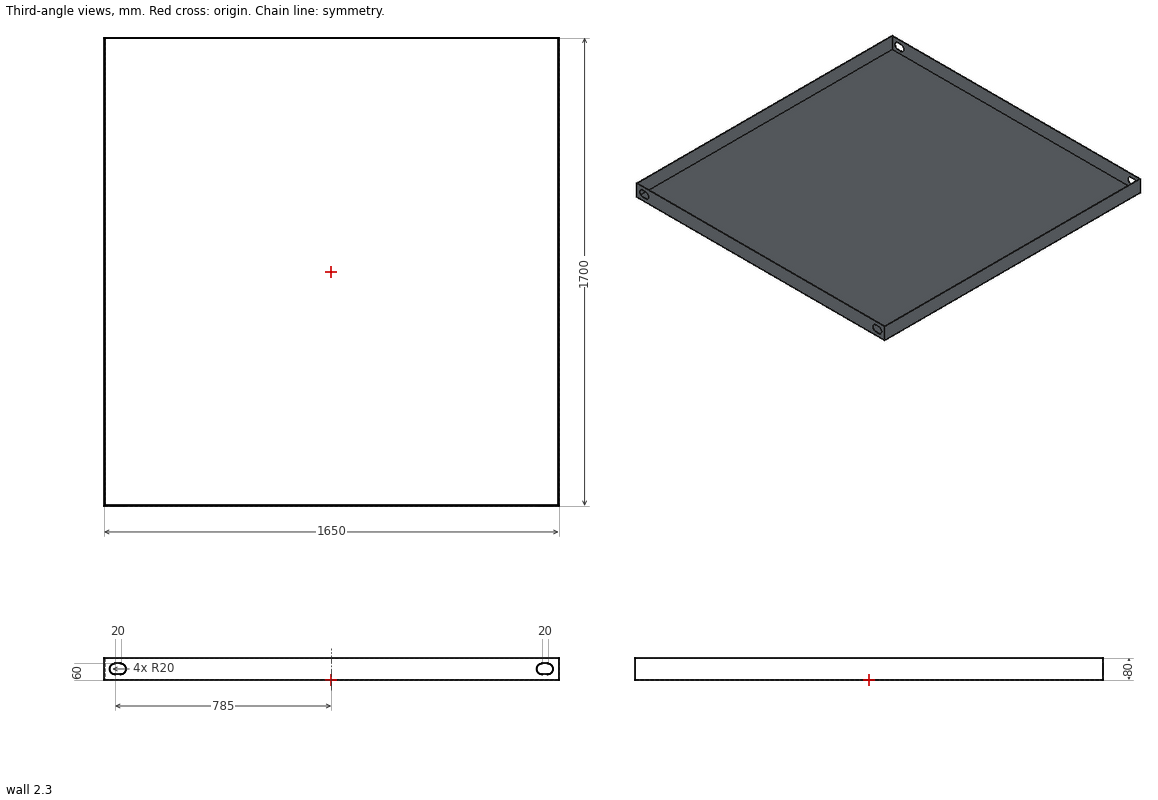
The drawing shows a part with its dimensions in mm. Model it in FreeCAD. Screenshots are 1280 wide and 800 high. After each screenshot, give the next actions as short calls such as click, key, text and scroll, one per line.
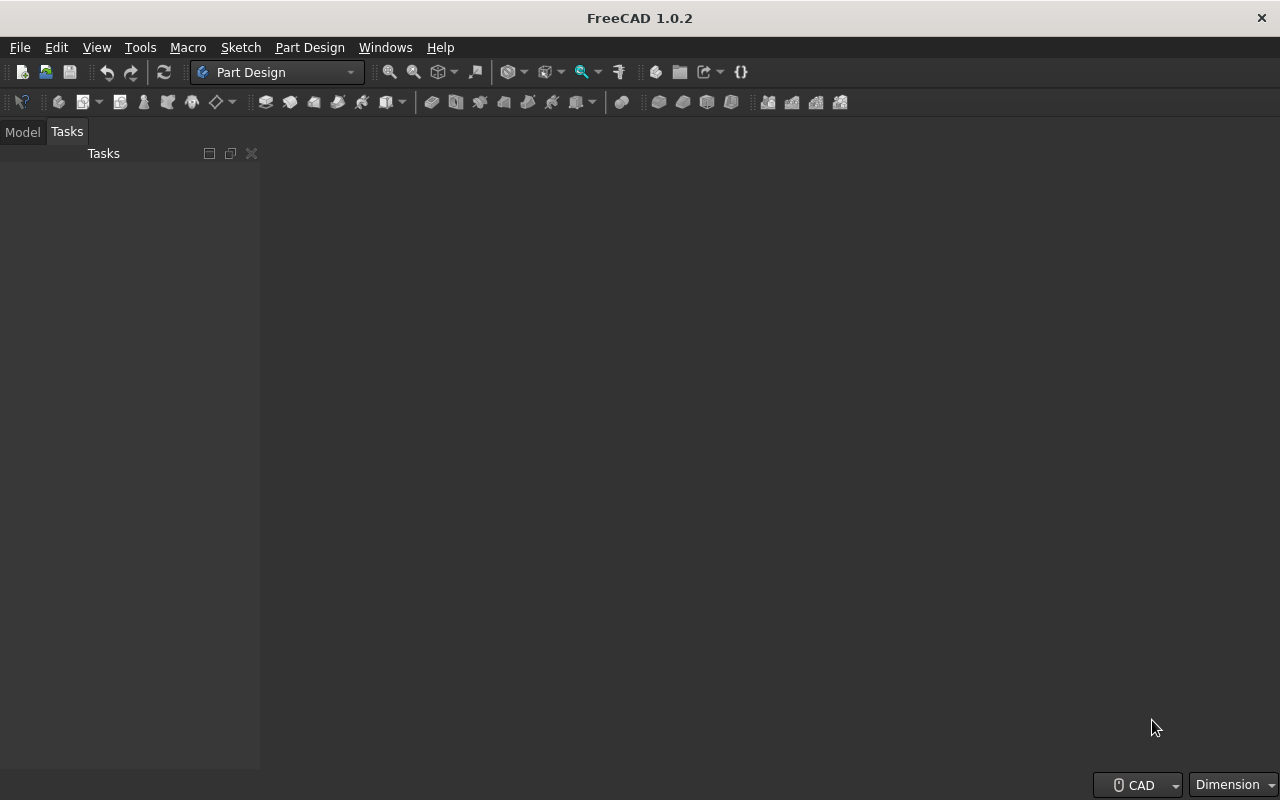
key(ctrl+n)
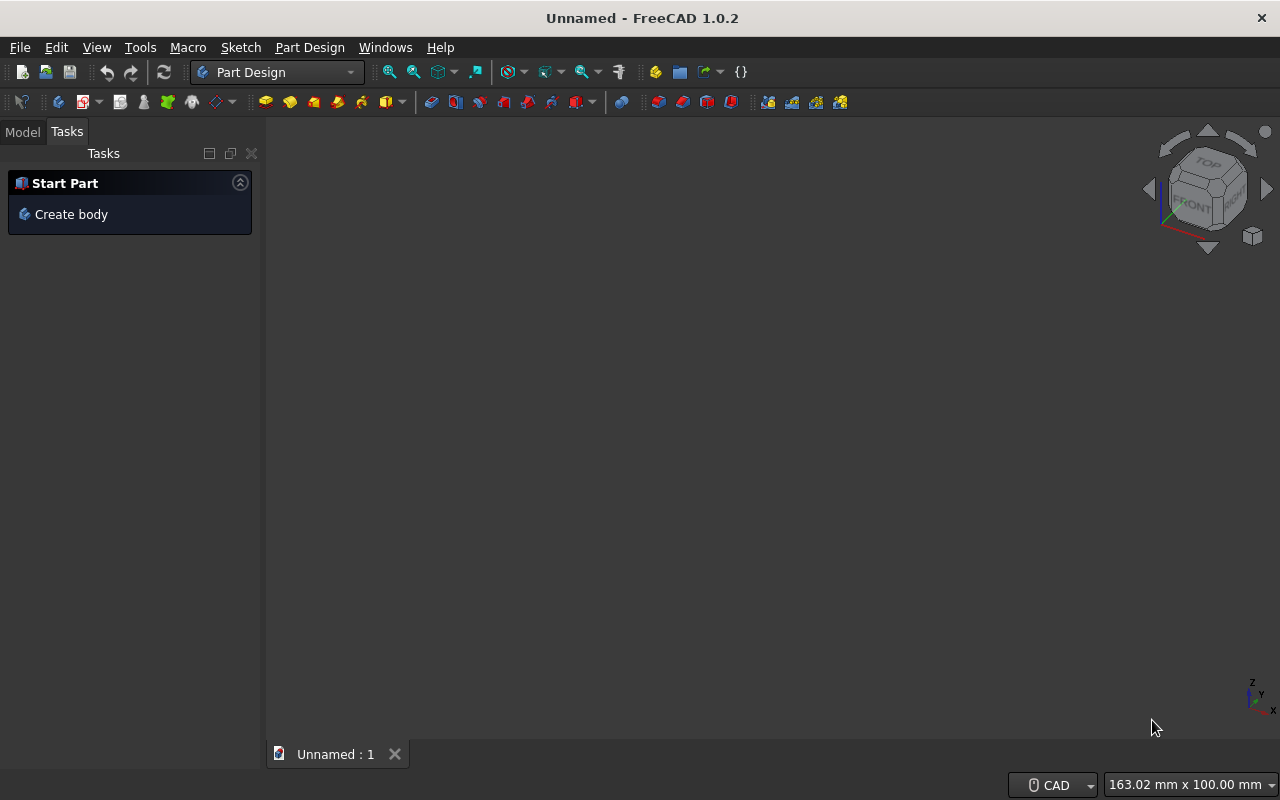
click(84, 102)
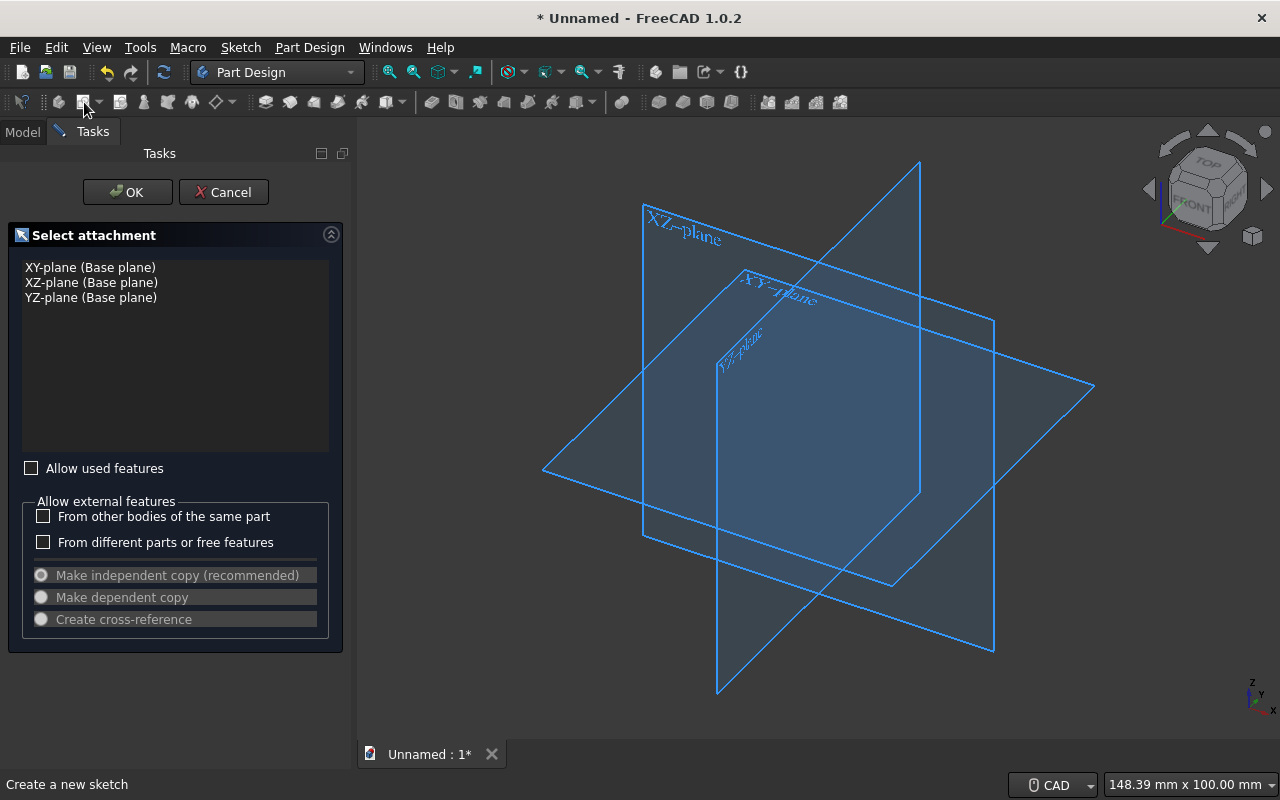
click(82, 268)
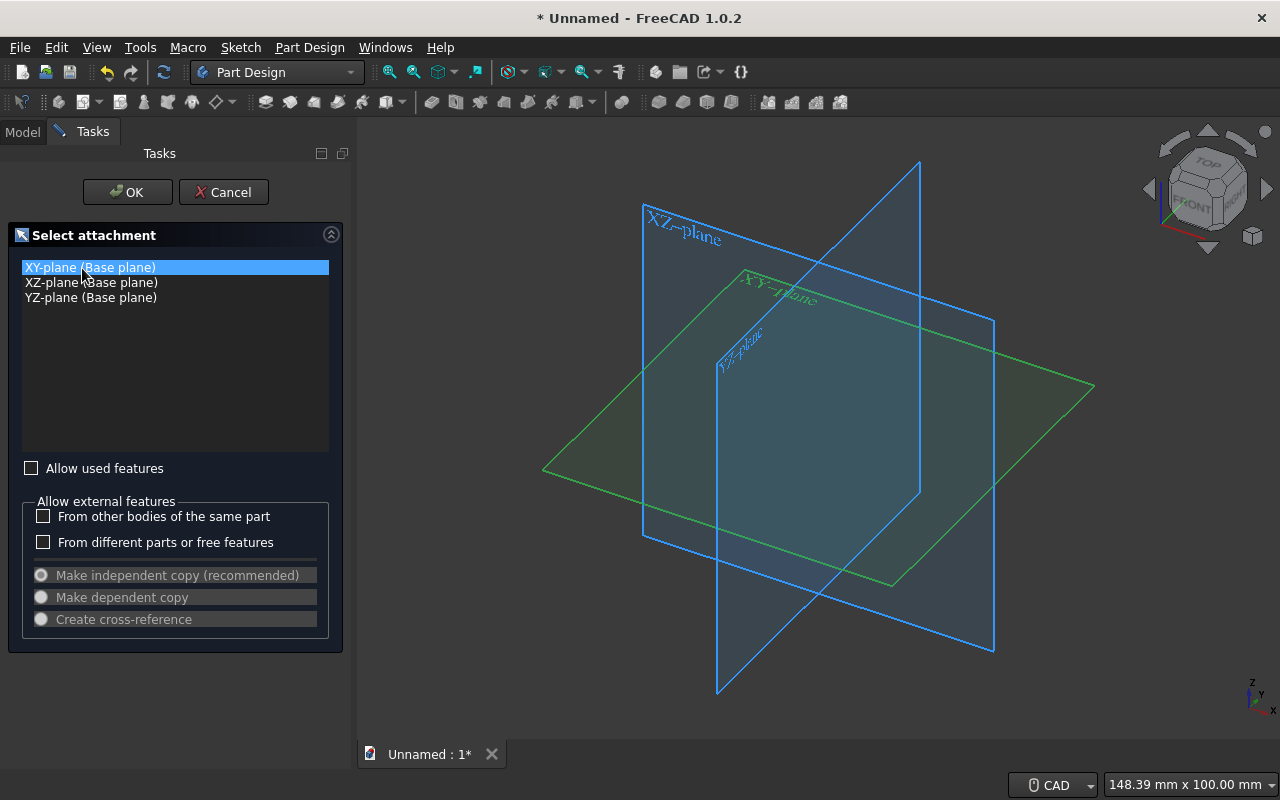
click(128, 192)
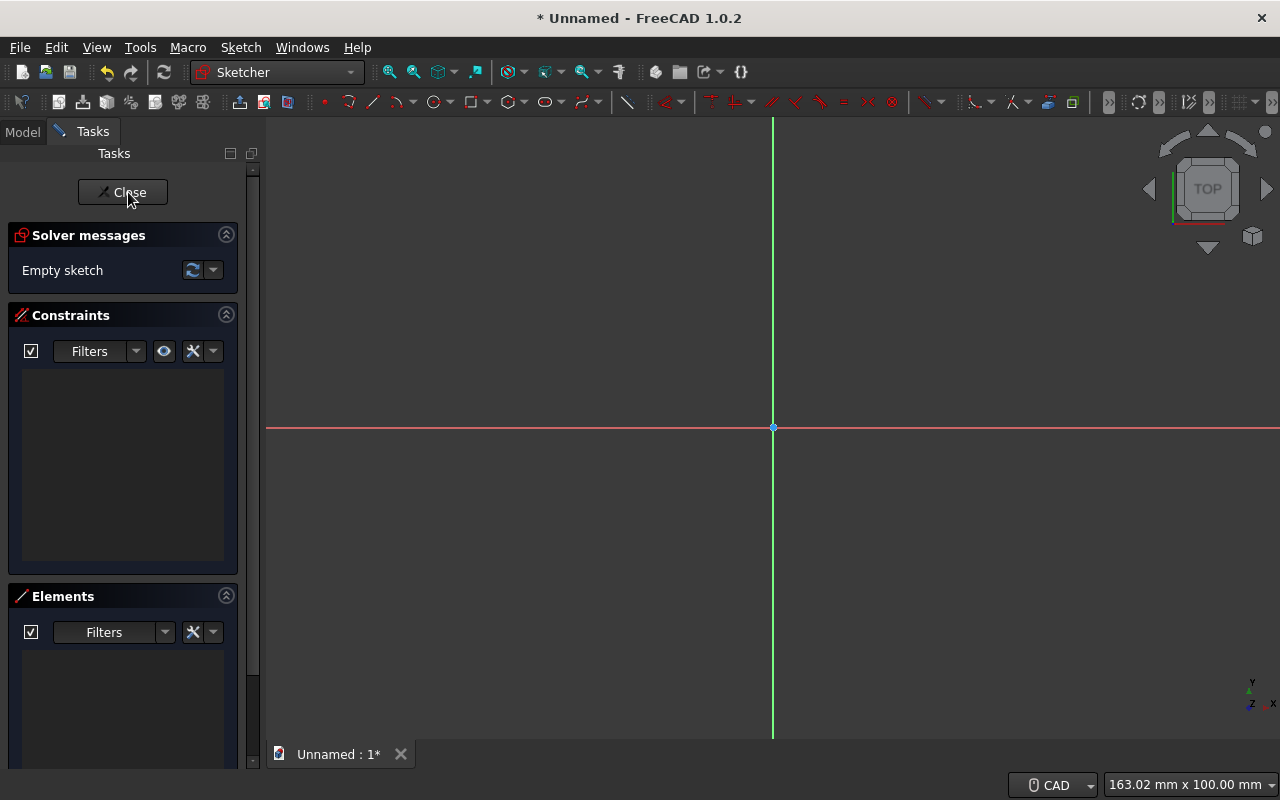
scroll(702, 428, down, 16)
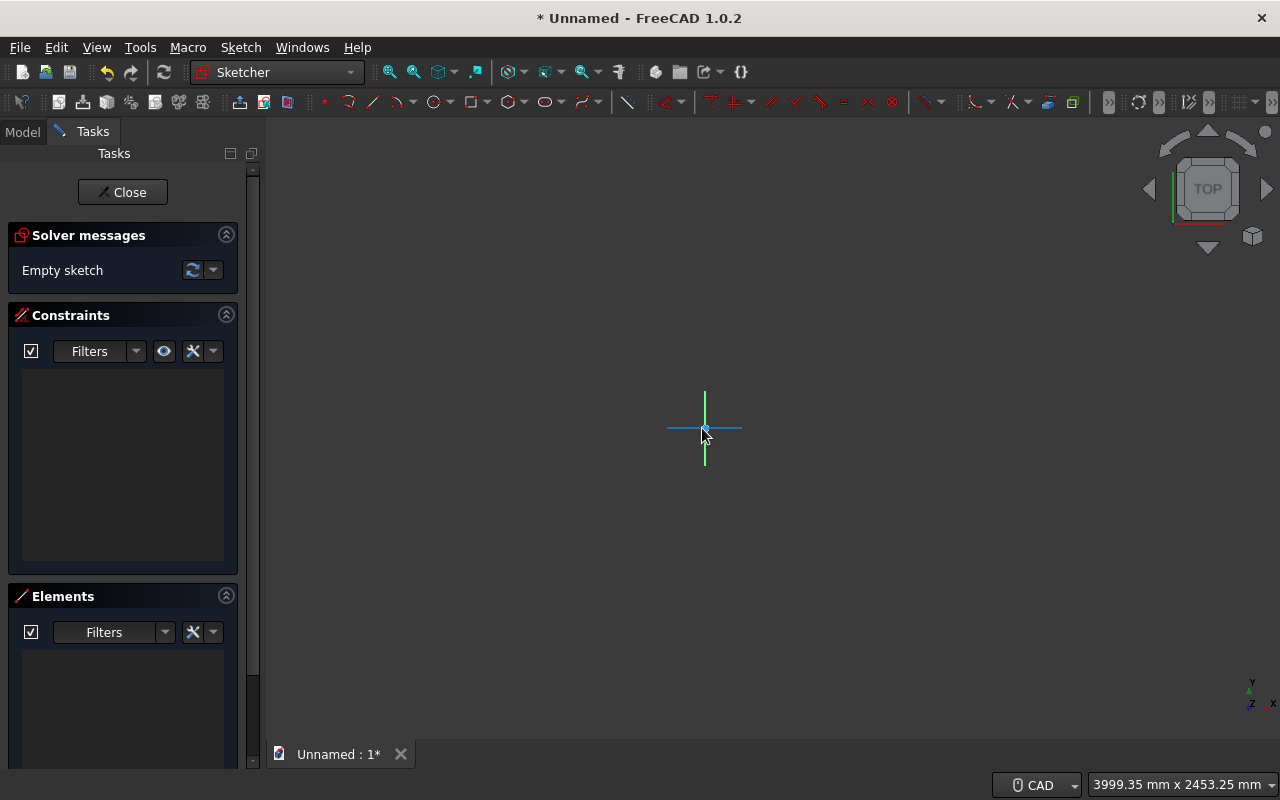
key(g)
key(v)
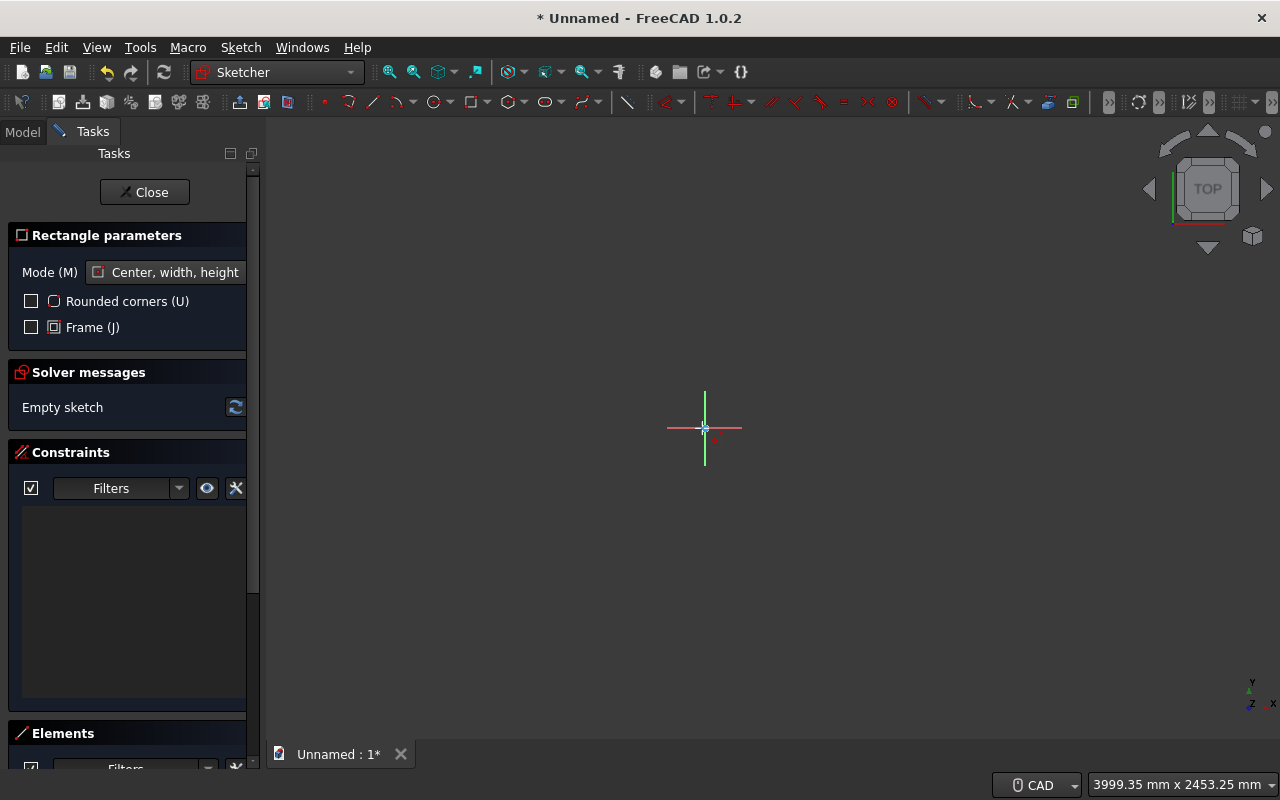
click(705, 428)
move(914, 213)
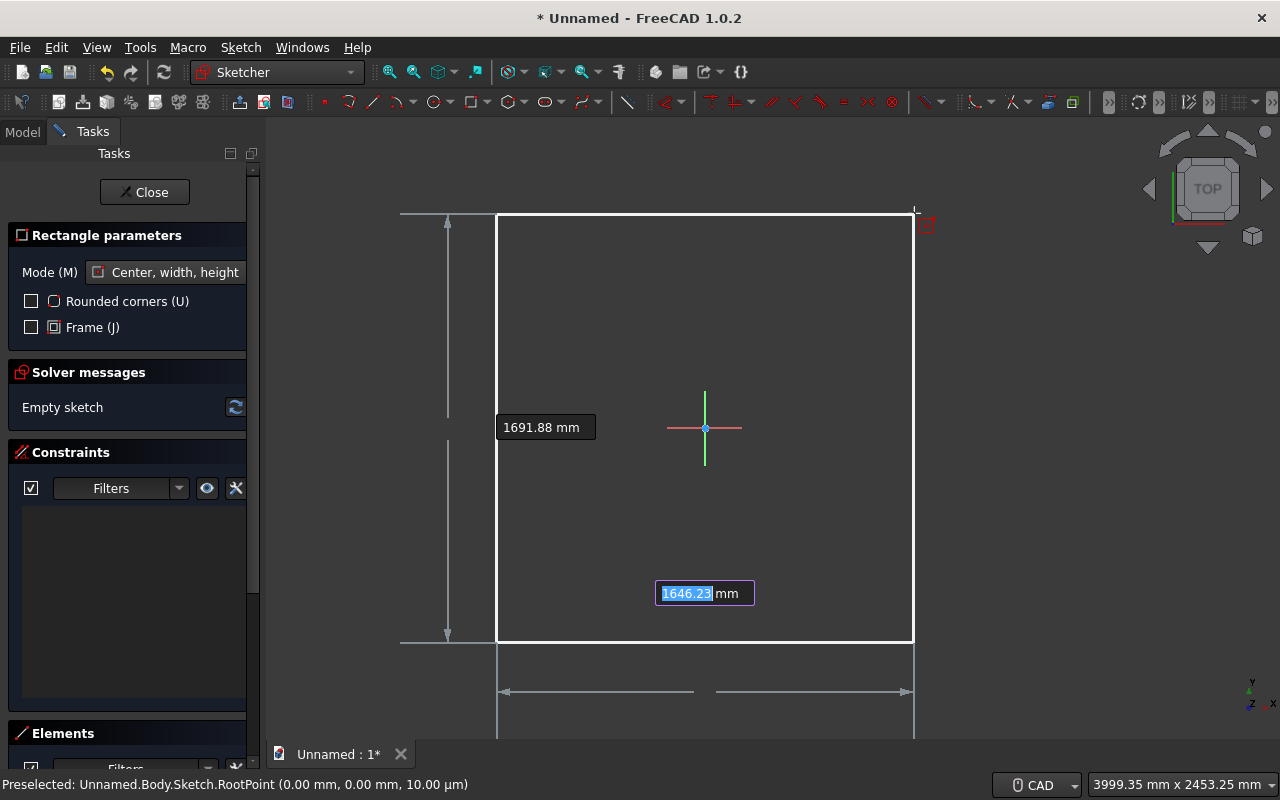
text(1650)
key(Tab)
text(1700)
key(Return)
key(Escape)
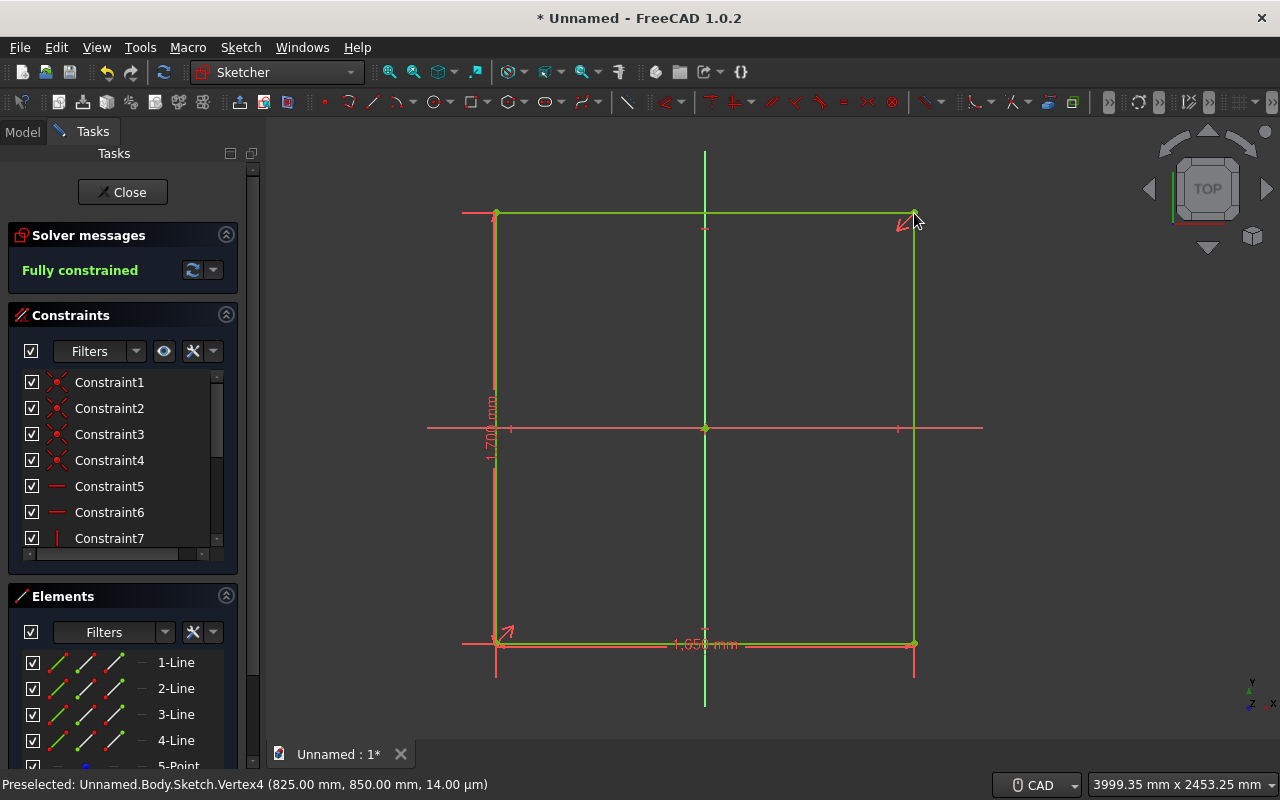
click(123, 192)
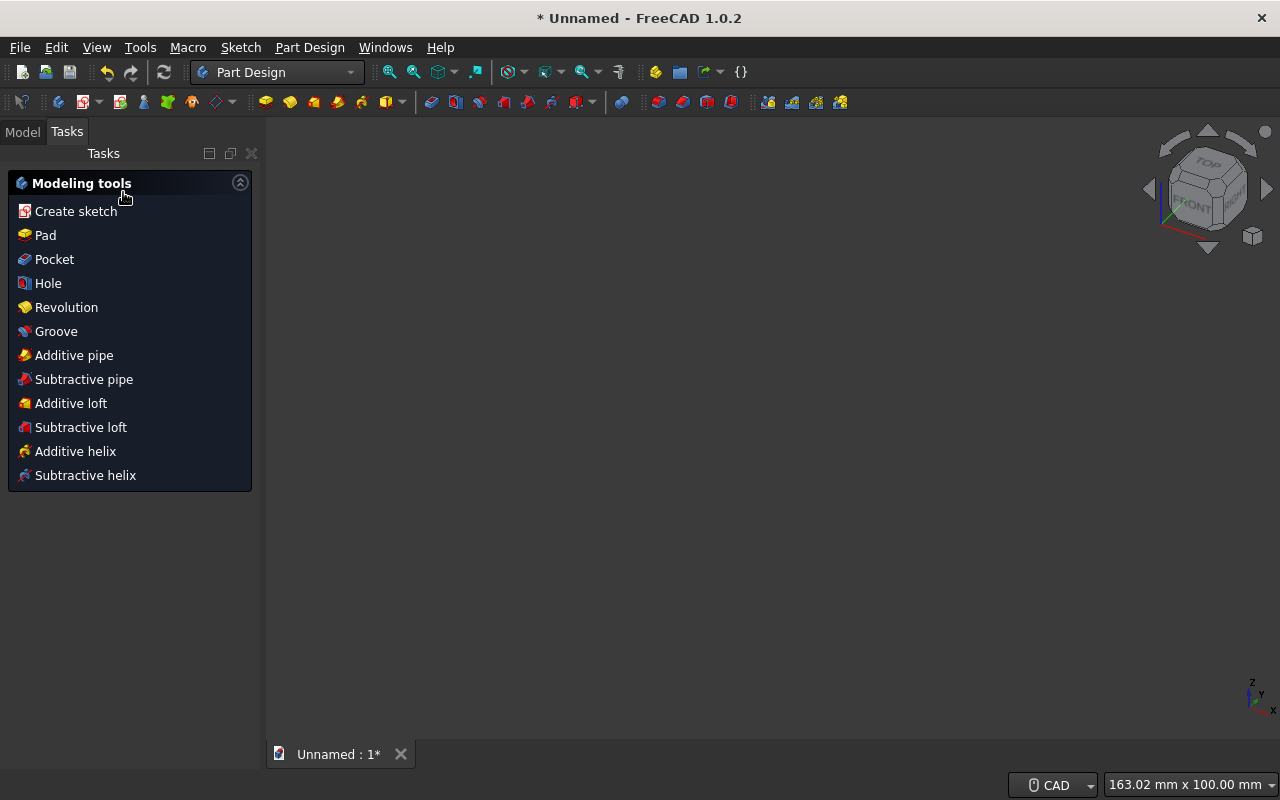
click(266, 102)